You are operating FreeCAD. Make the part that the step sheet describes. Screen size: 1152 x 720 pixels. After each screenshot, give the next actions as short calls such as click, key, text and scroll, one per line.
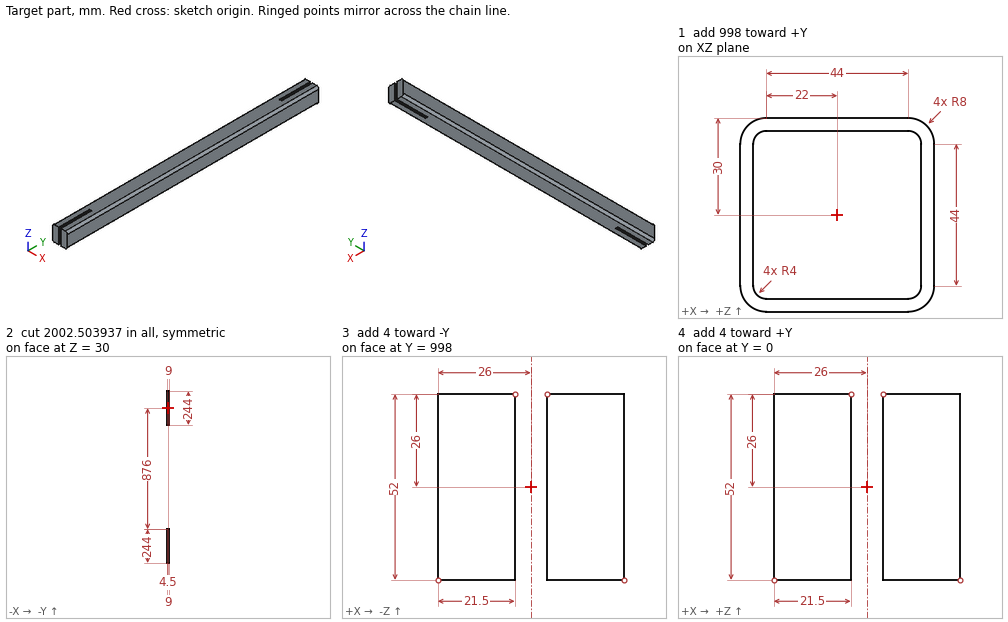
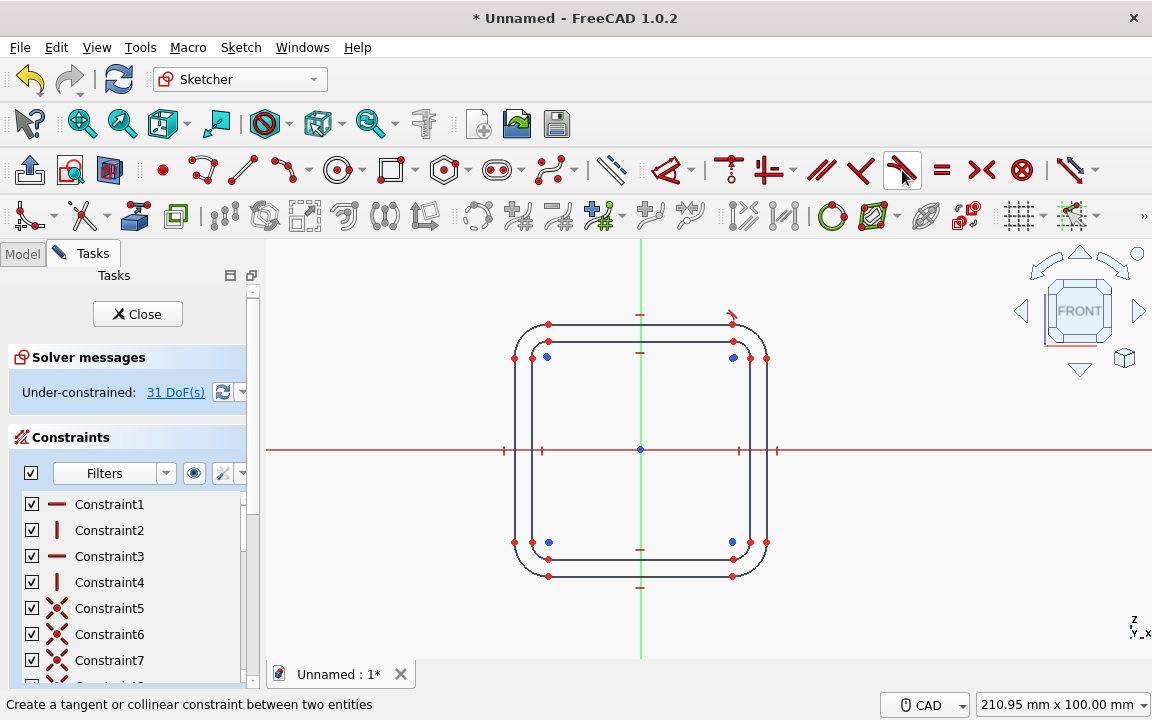
click(604, 325)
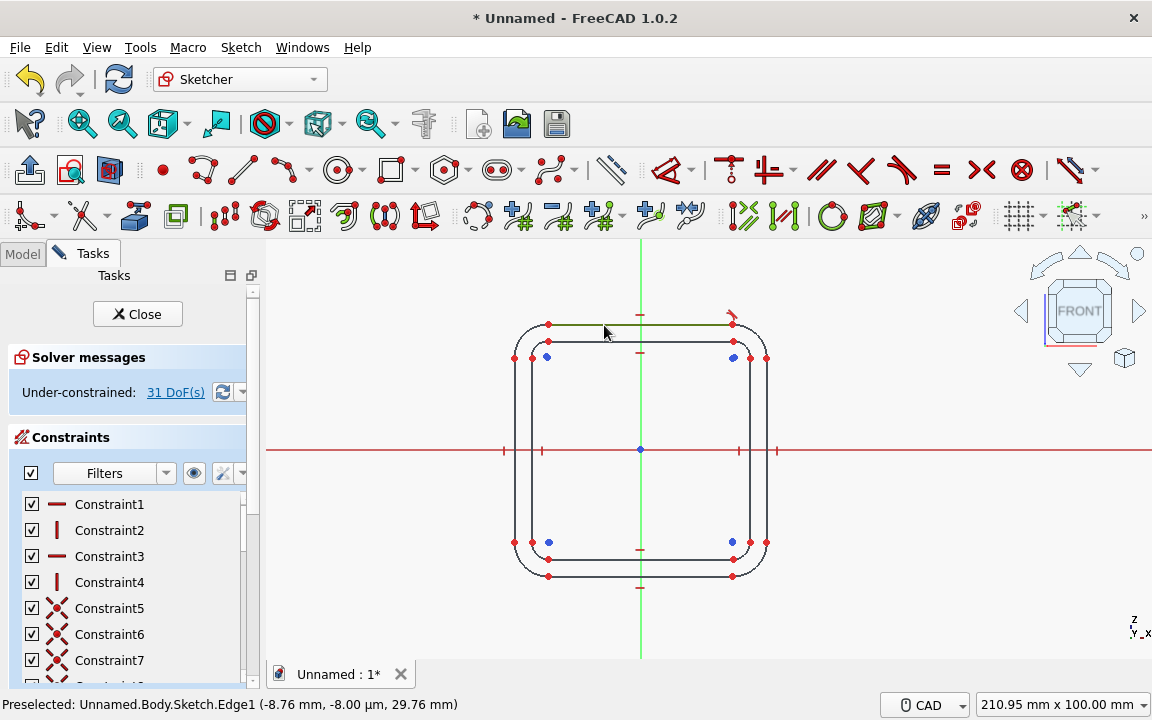
click(533, 328)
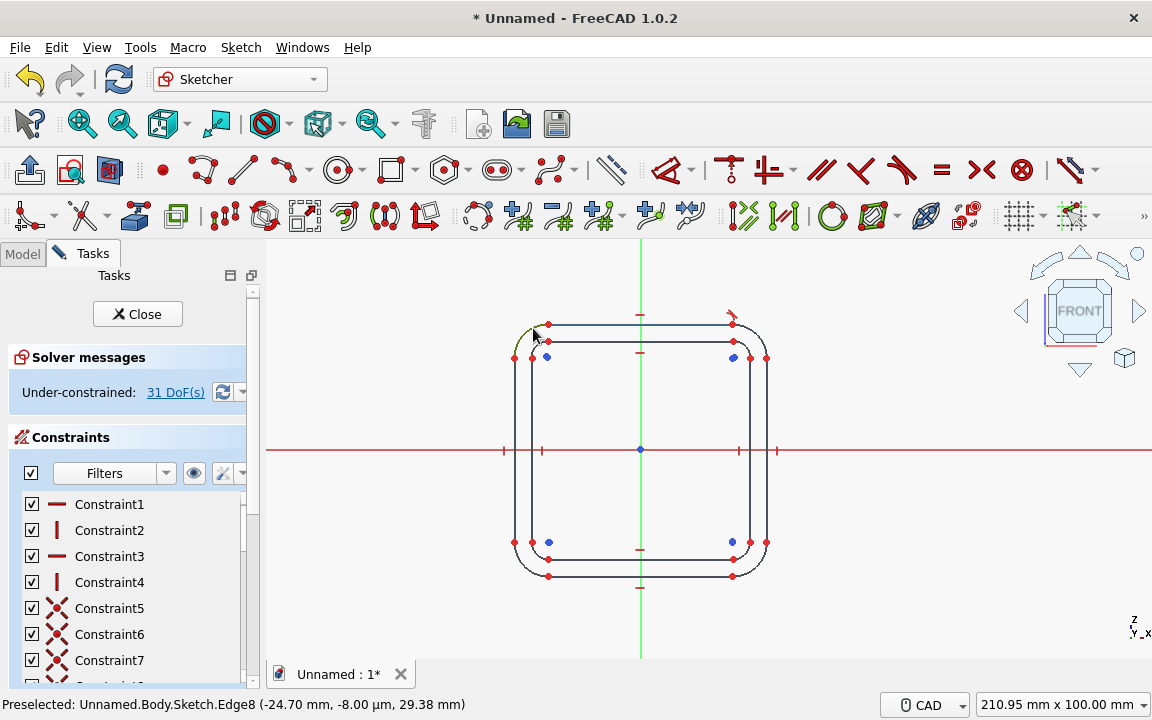
click(902, 170)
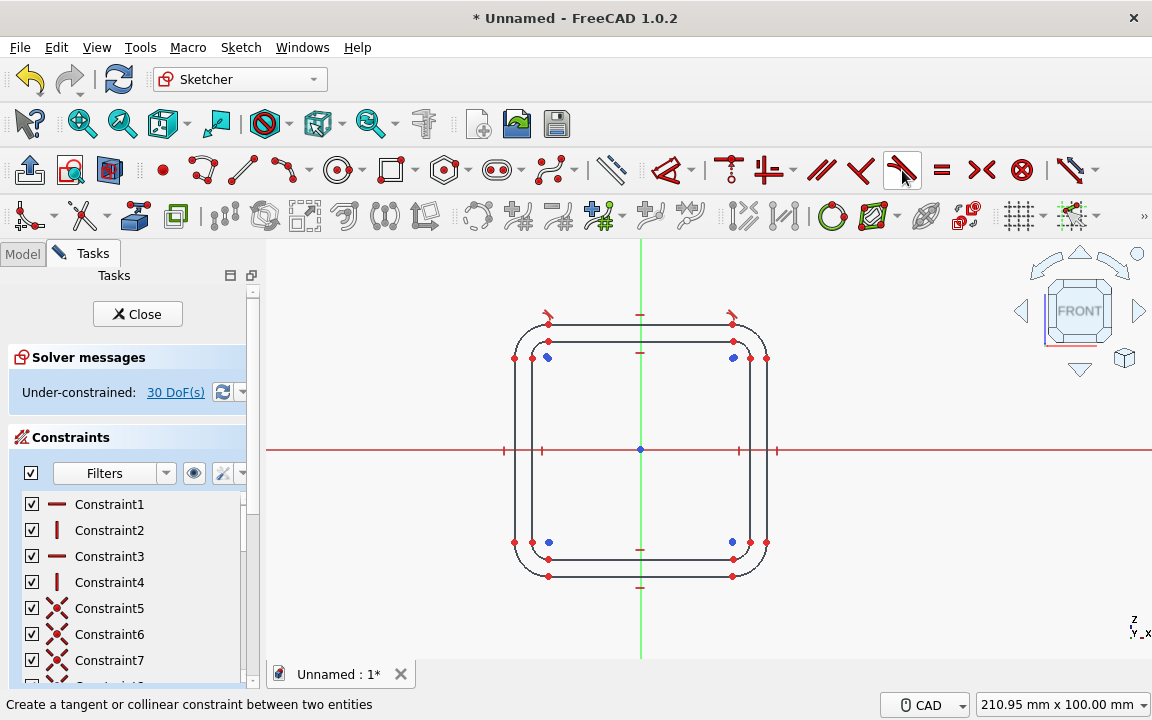
click(767, 414)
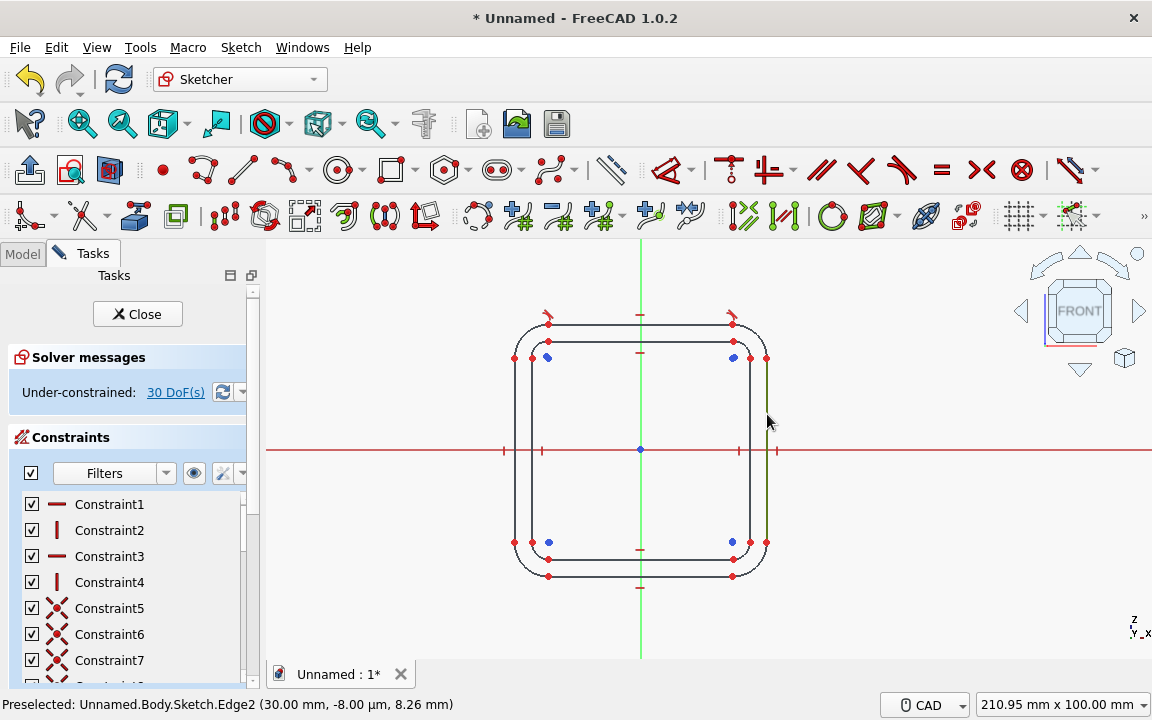
click(763, 343)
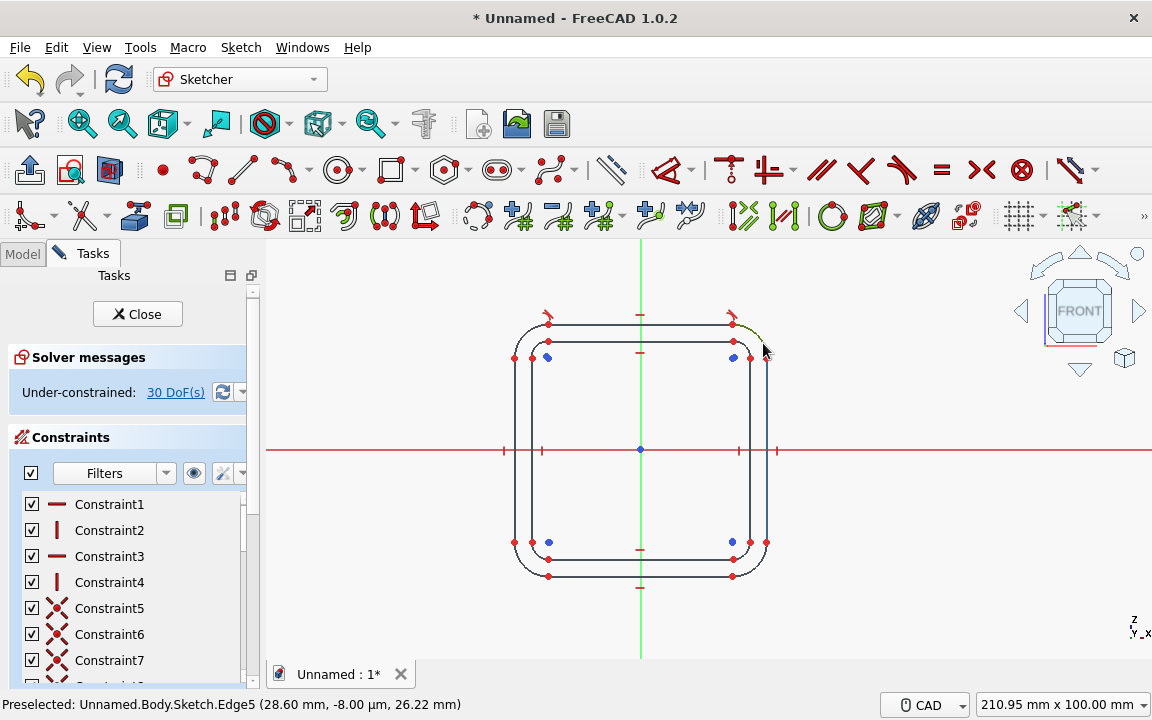
click(902, 170)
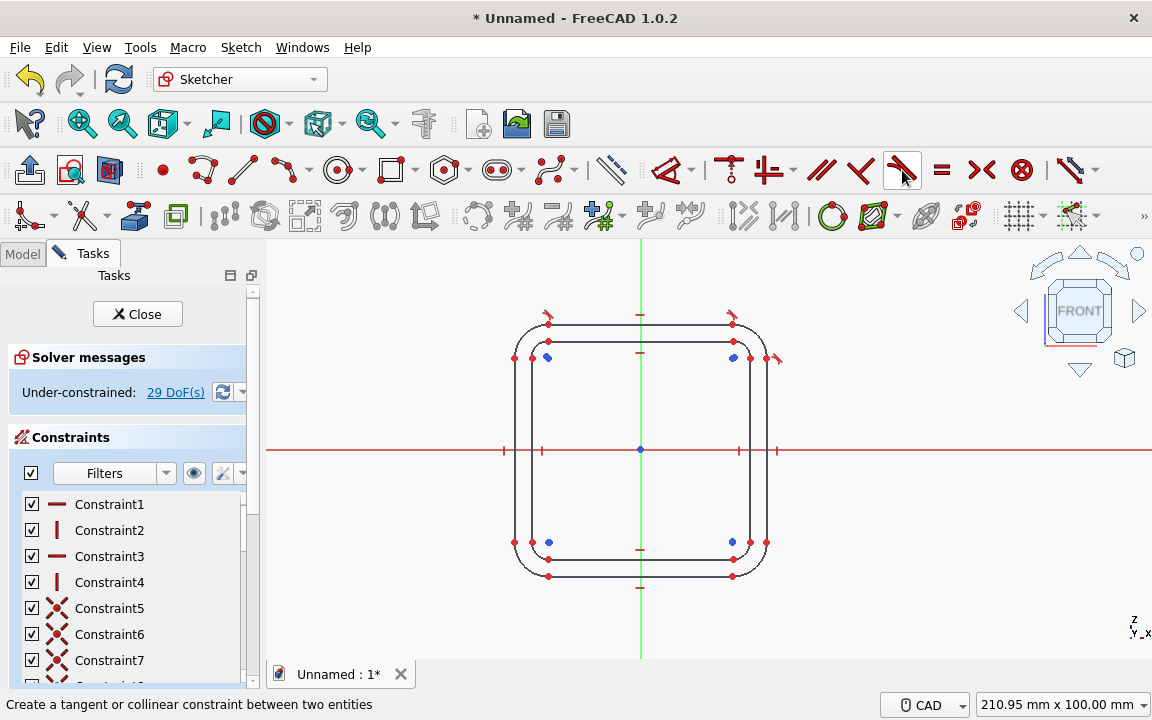
click(767, 414)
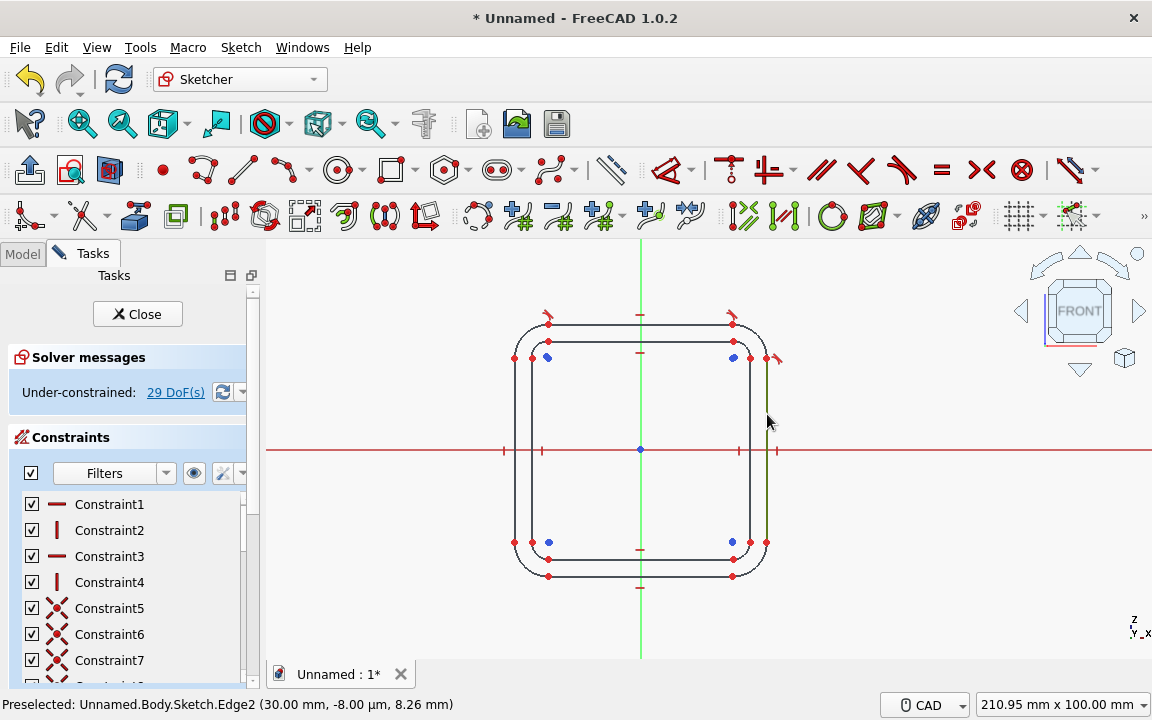
click(748, 573)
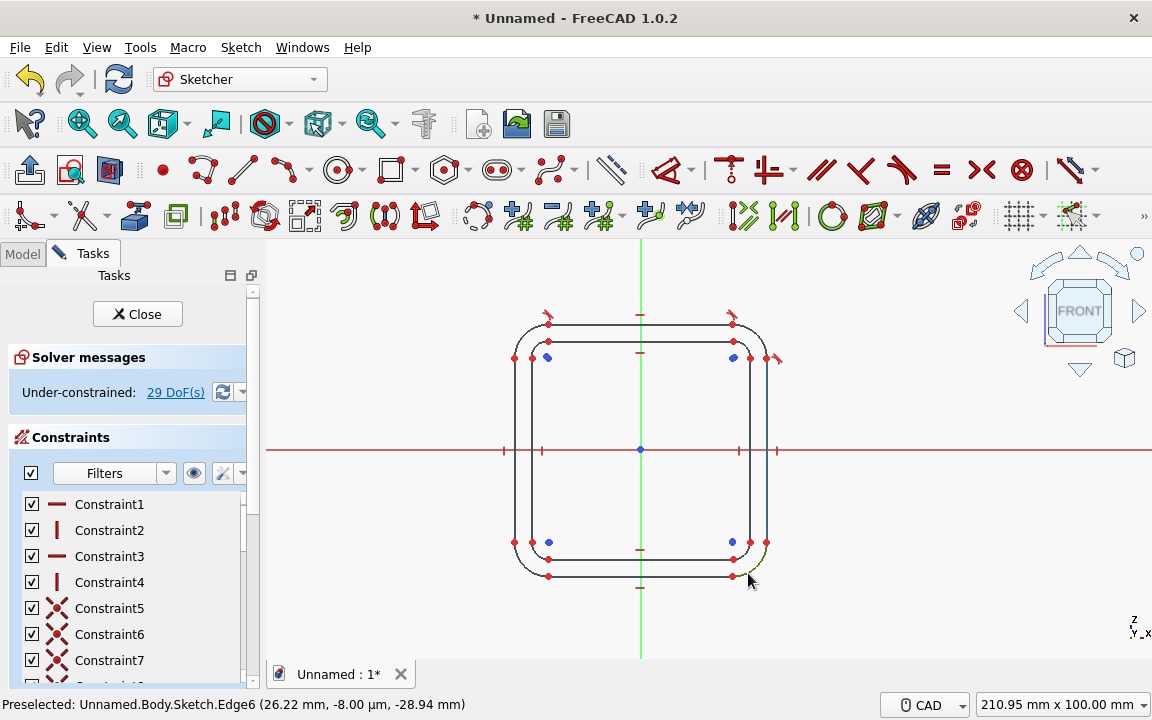
click(902, 170)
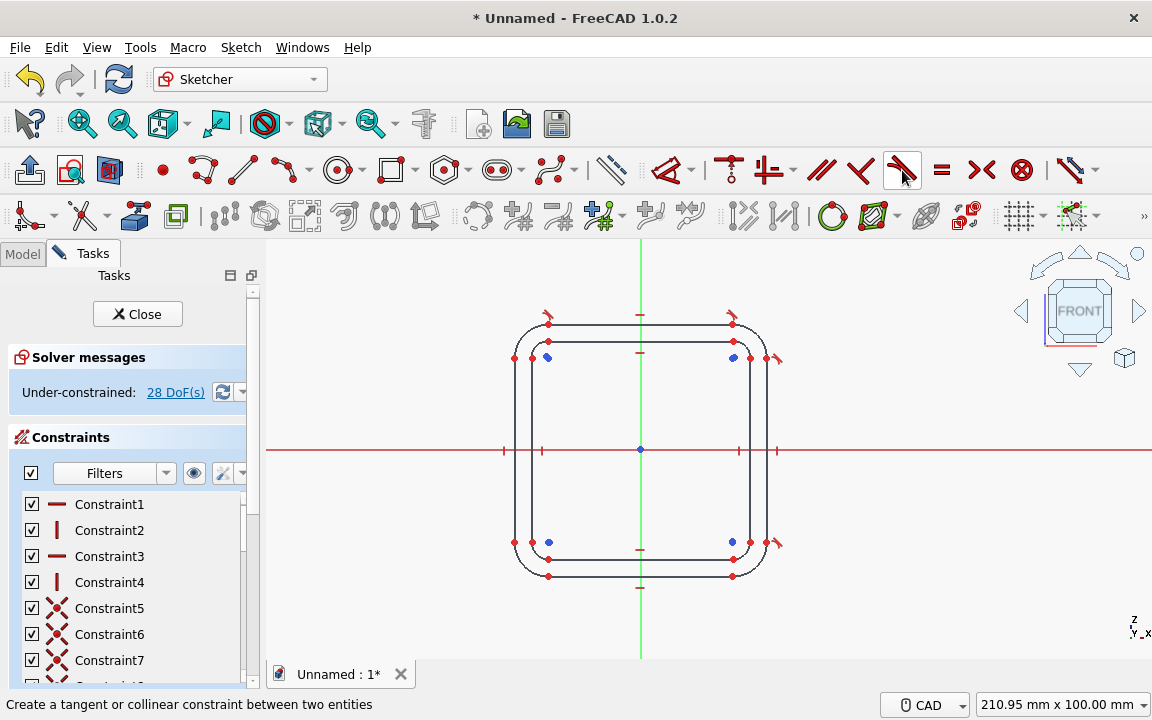
click(678, 577)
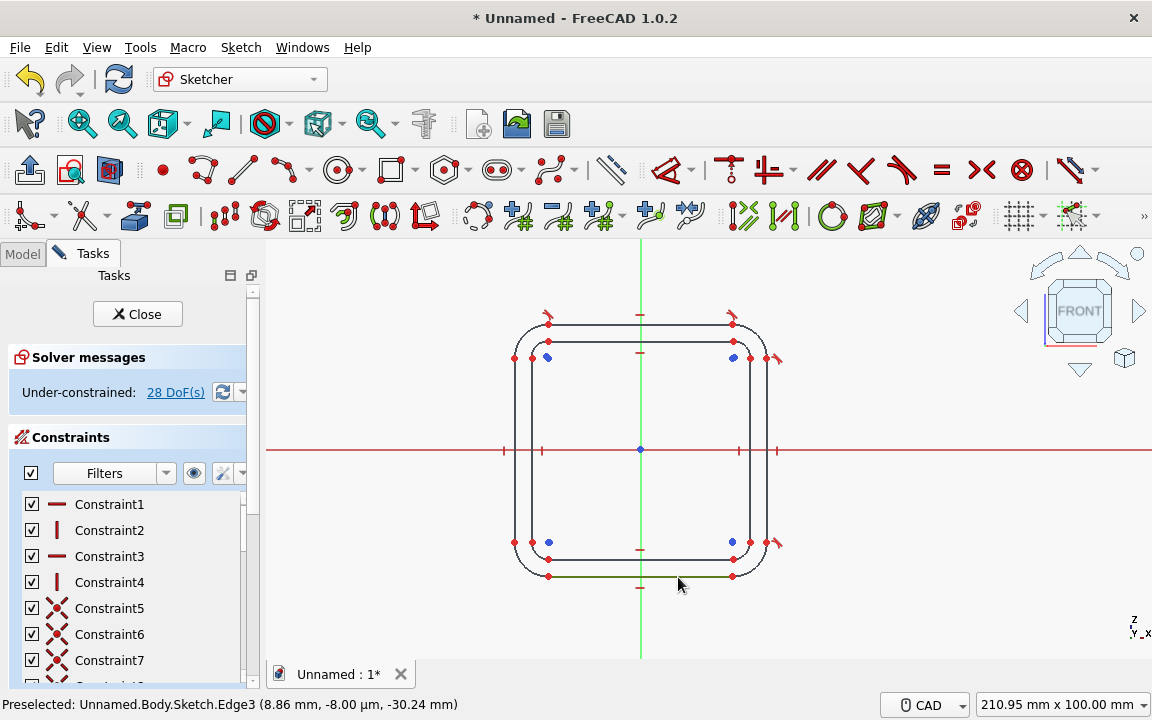
click(748, 573)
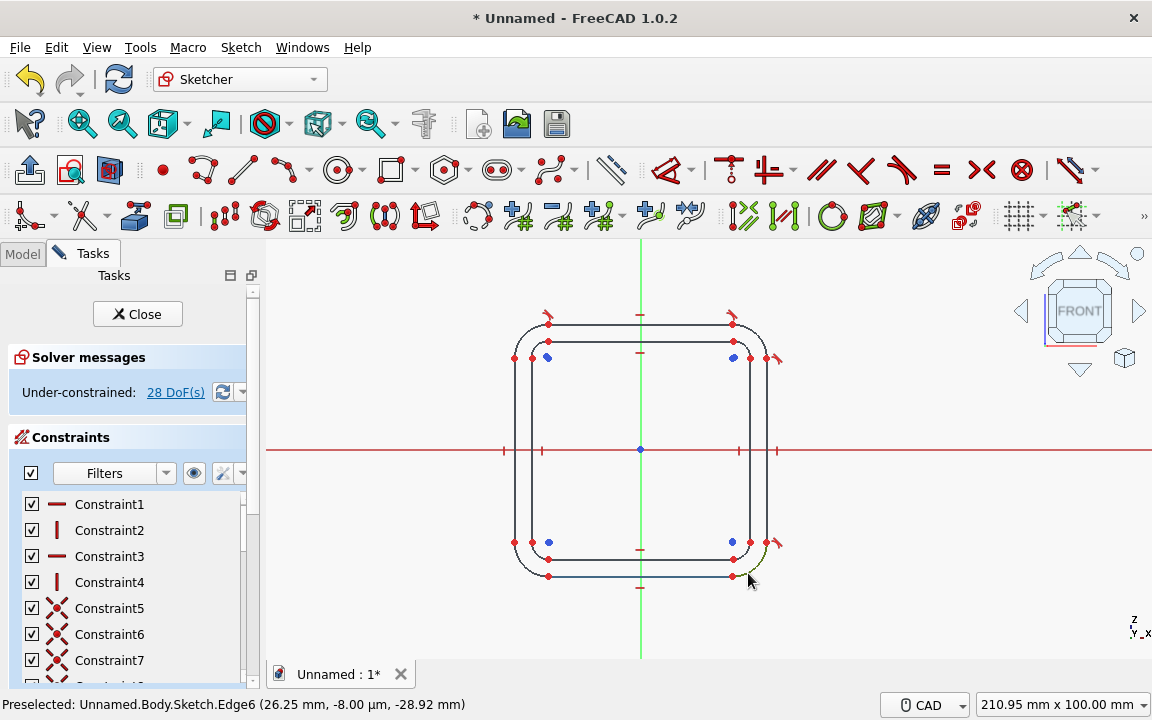
click(902, 170)